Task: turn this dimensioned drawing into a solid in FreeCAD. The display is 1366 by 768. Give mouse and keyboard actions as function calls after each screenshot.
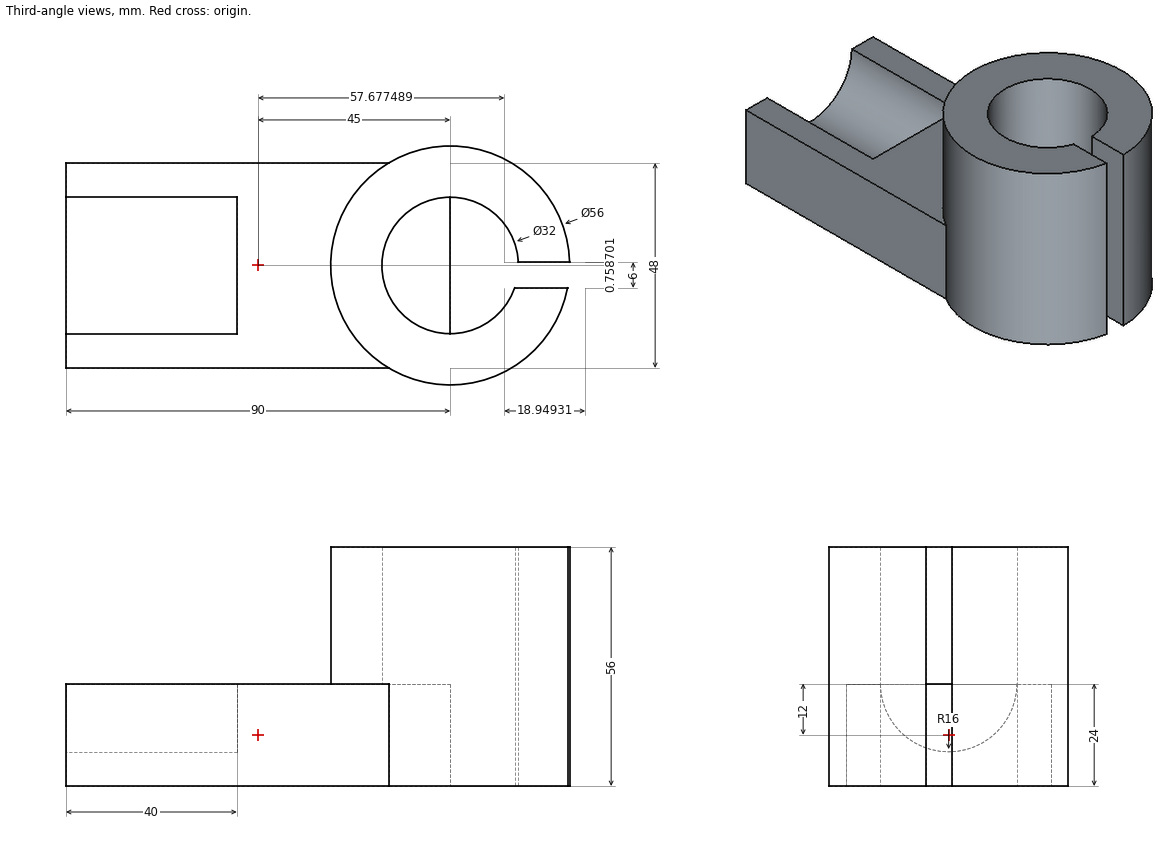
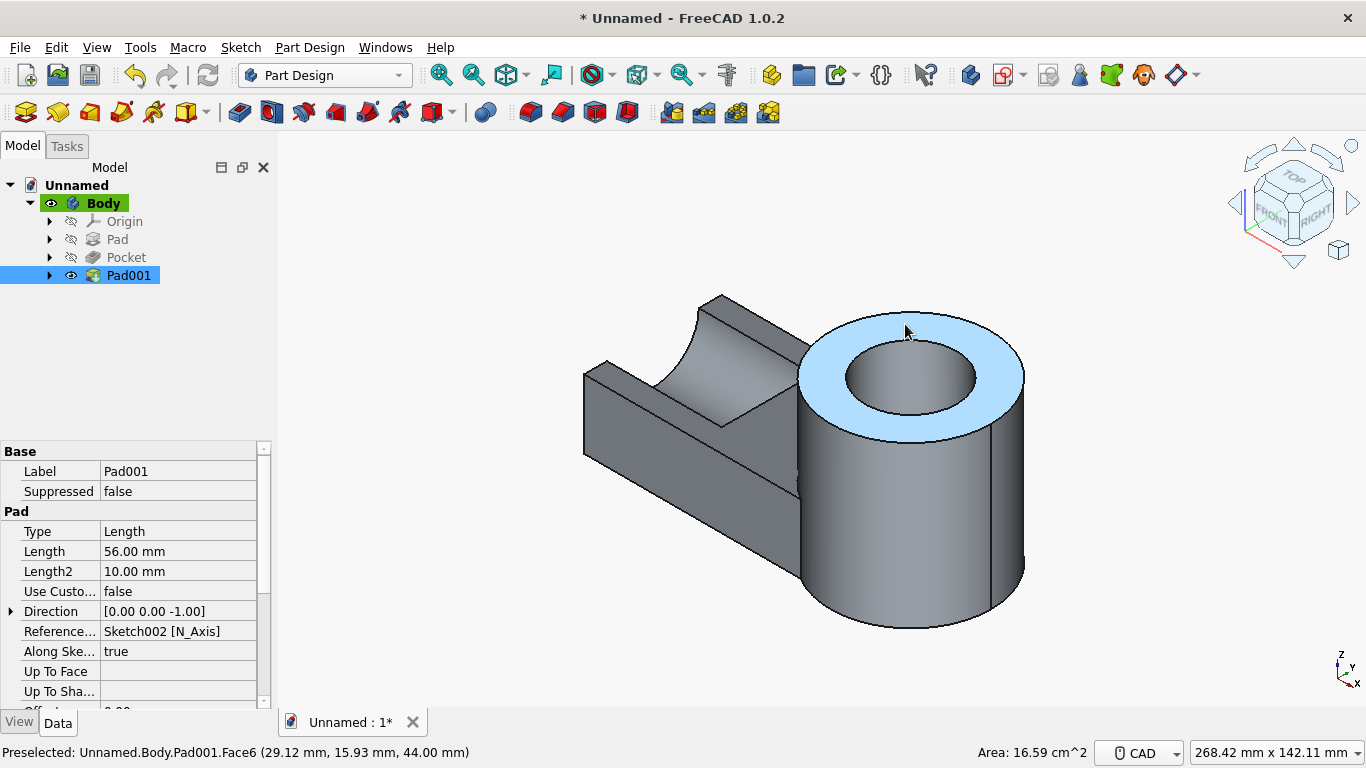
click(1004, 76)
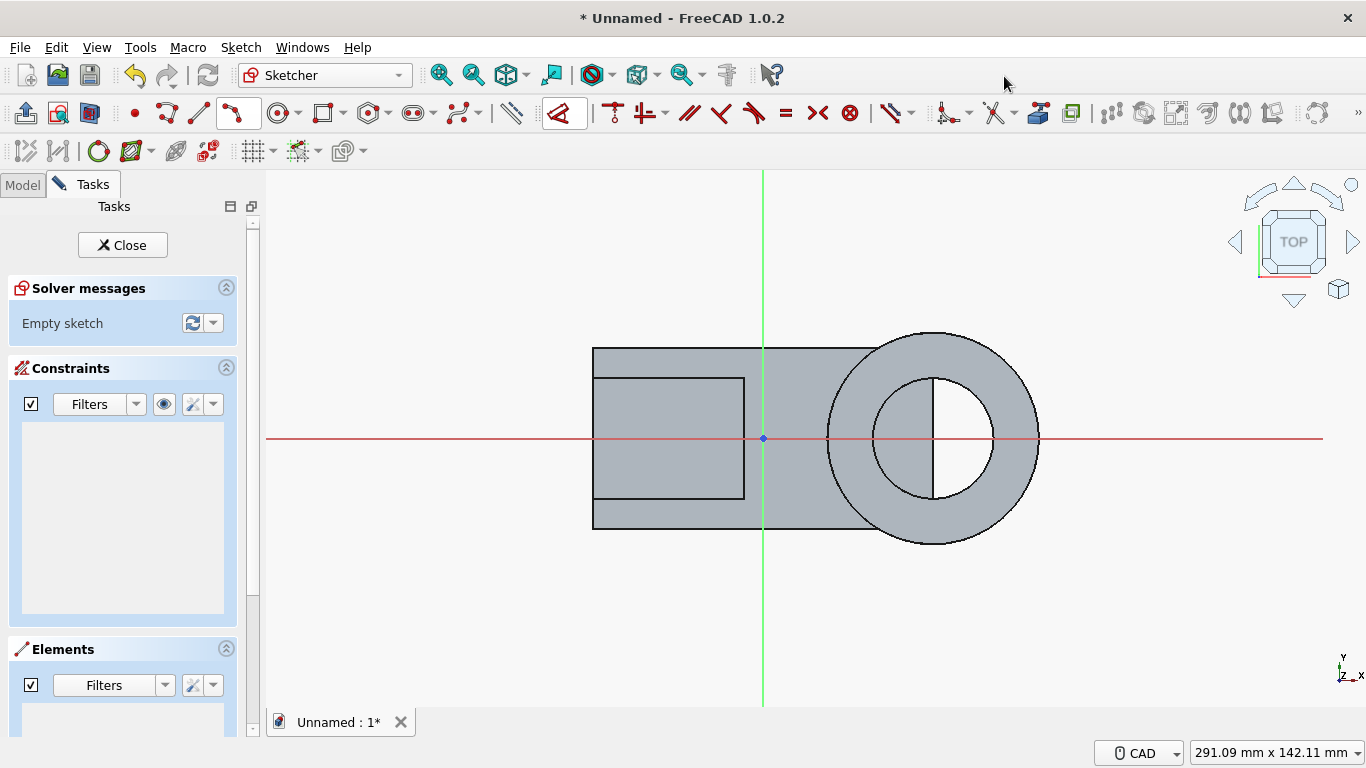
scroll(1050, 448, up, 11)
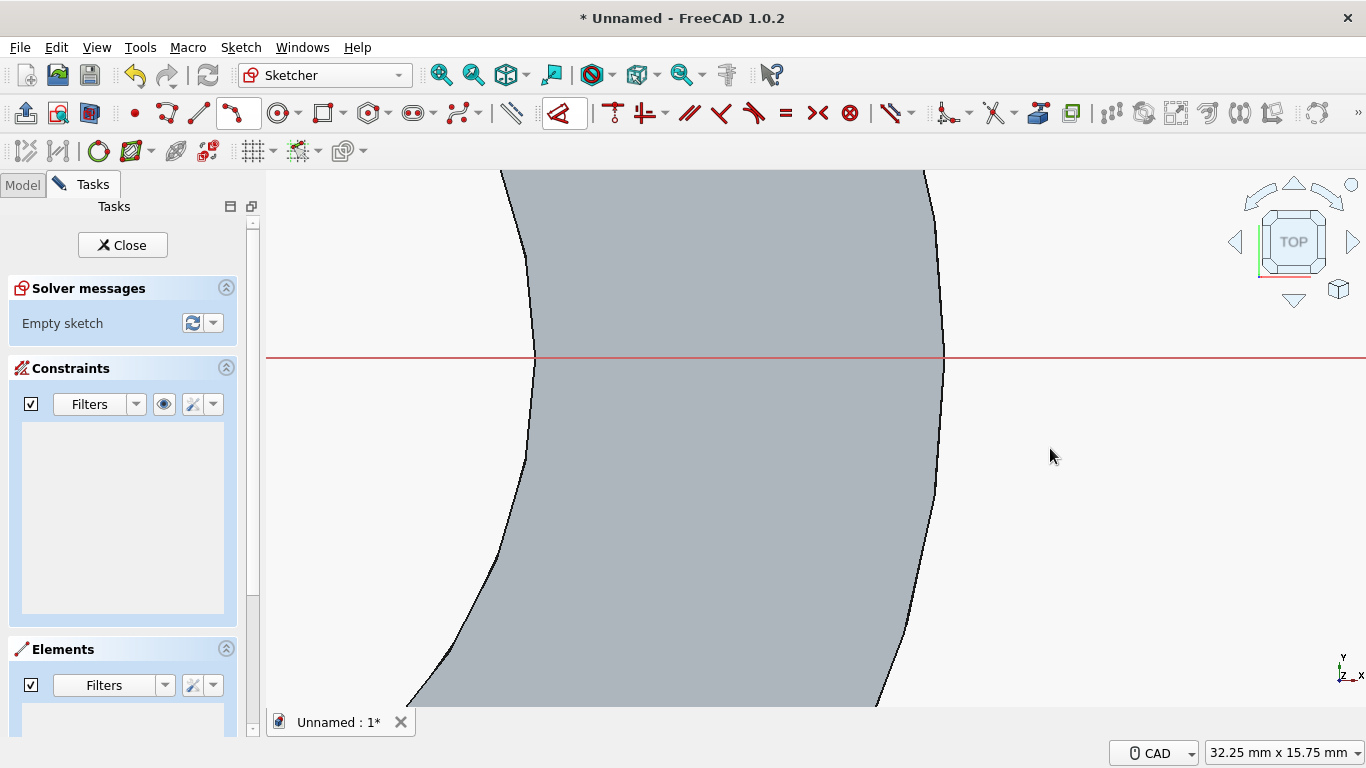
key(g)
key(r)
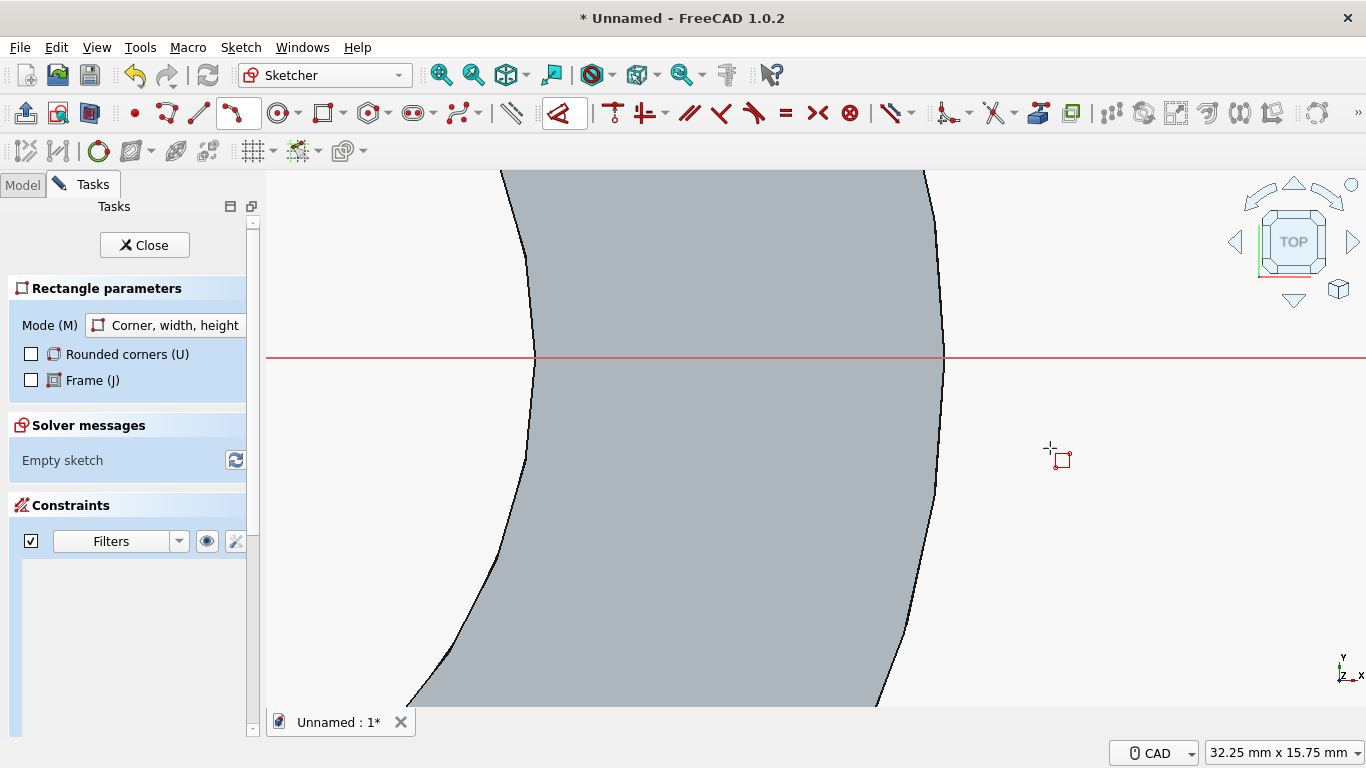
click(422, 332)
move(1068, 537)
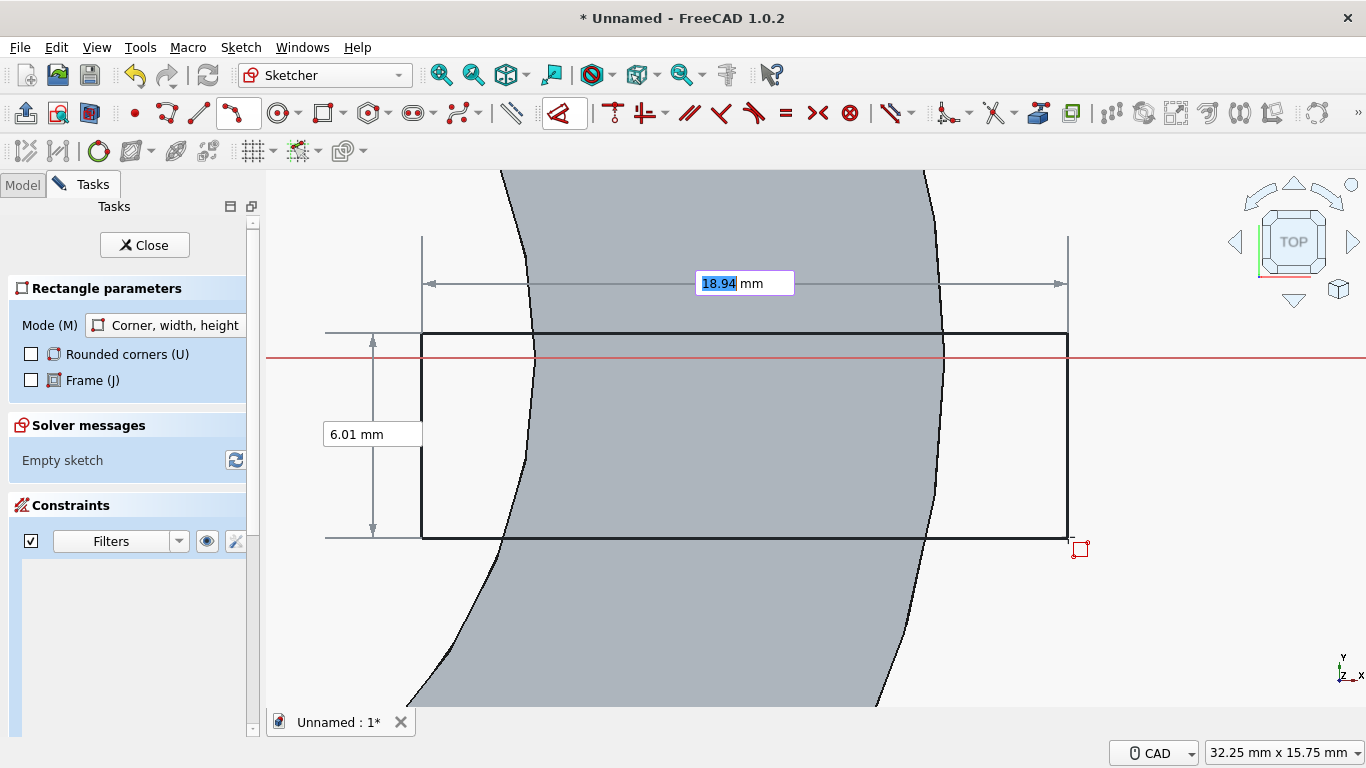
text(18.94931)
key(Tab)
text(6)
key(Return)
key(Escape)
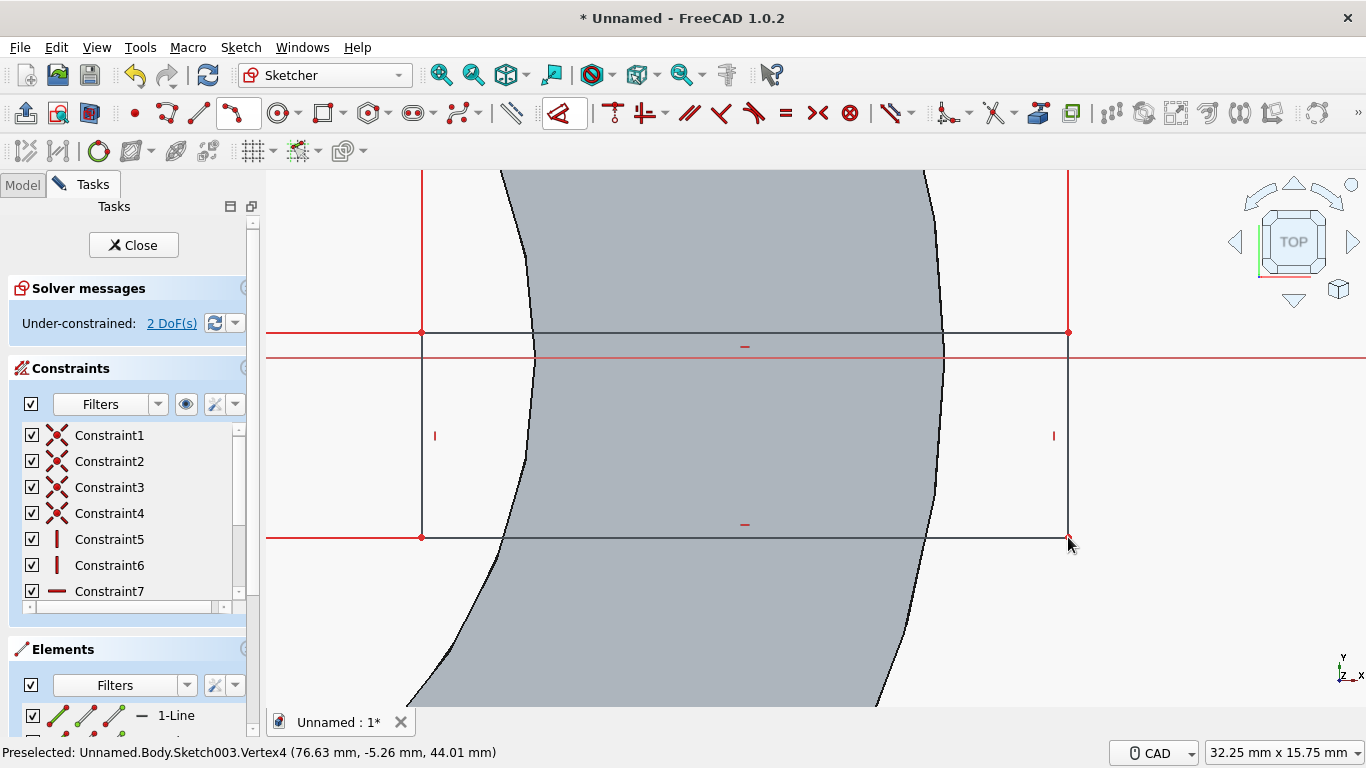
click(558, 114)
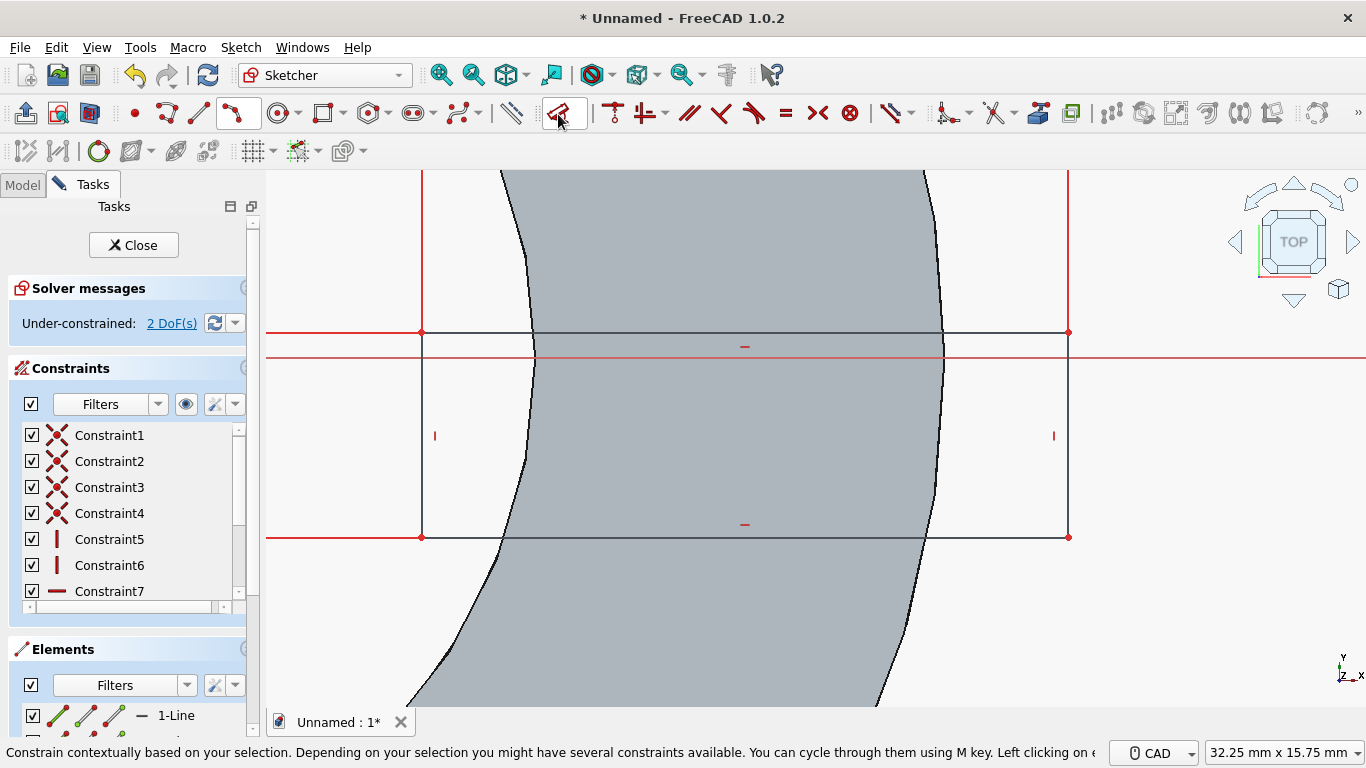
scroll(422, 333, up, 3)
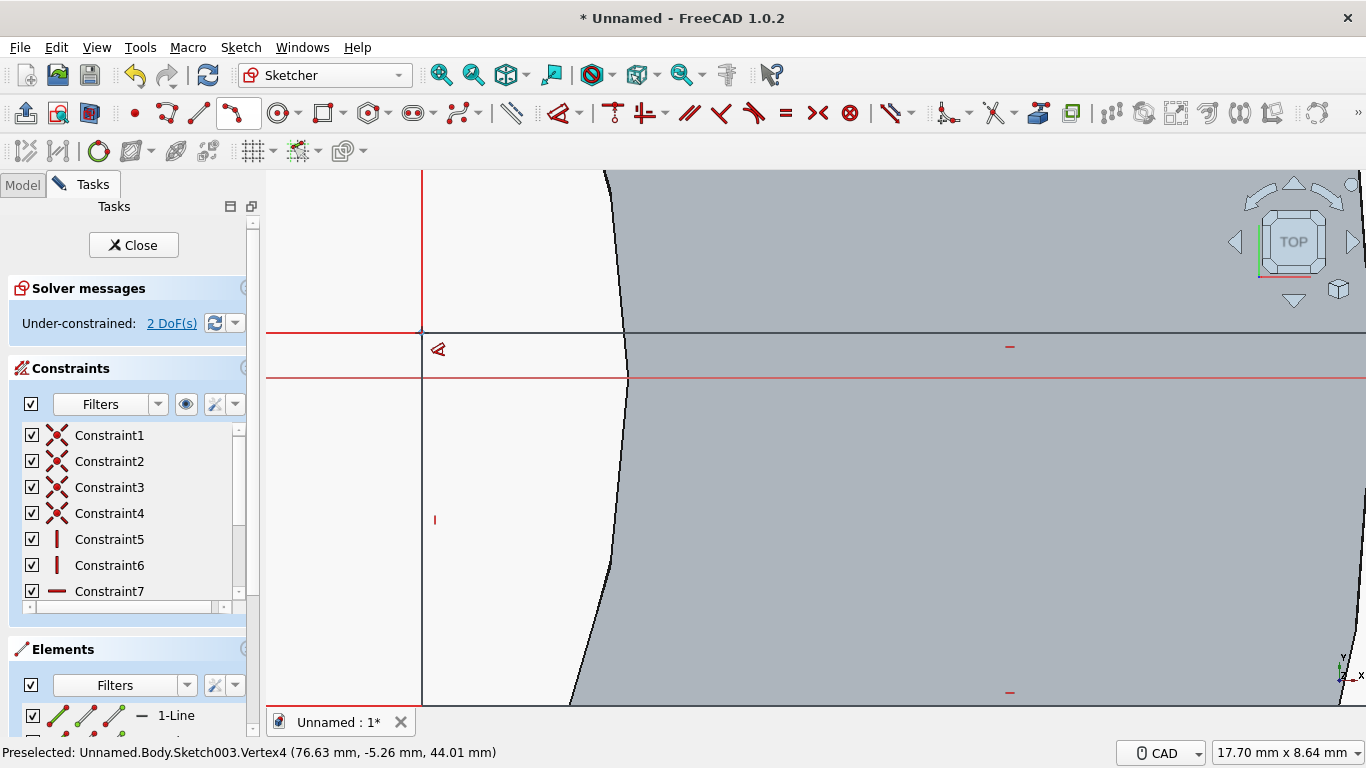
click(422, 333)
click(456, 356)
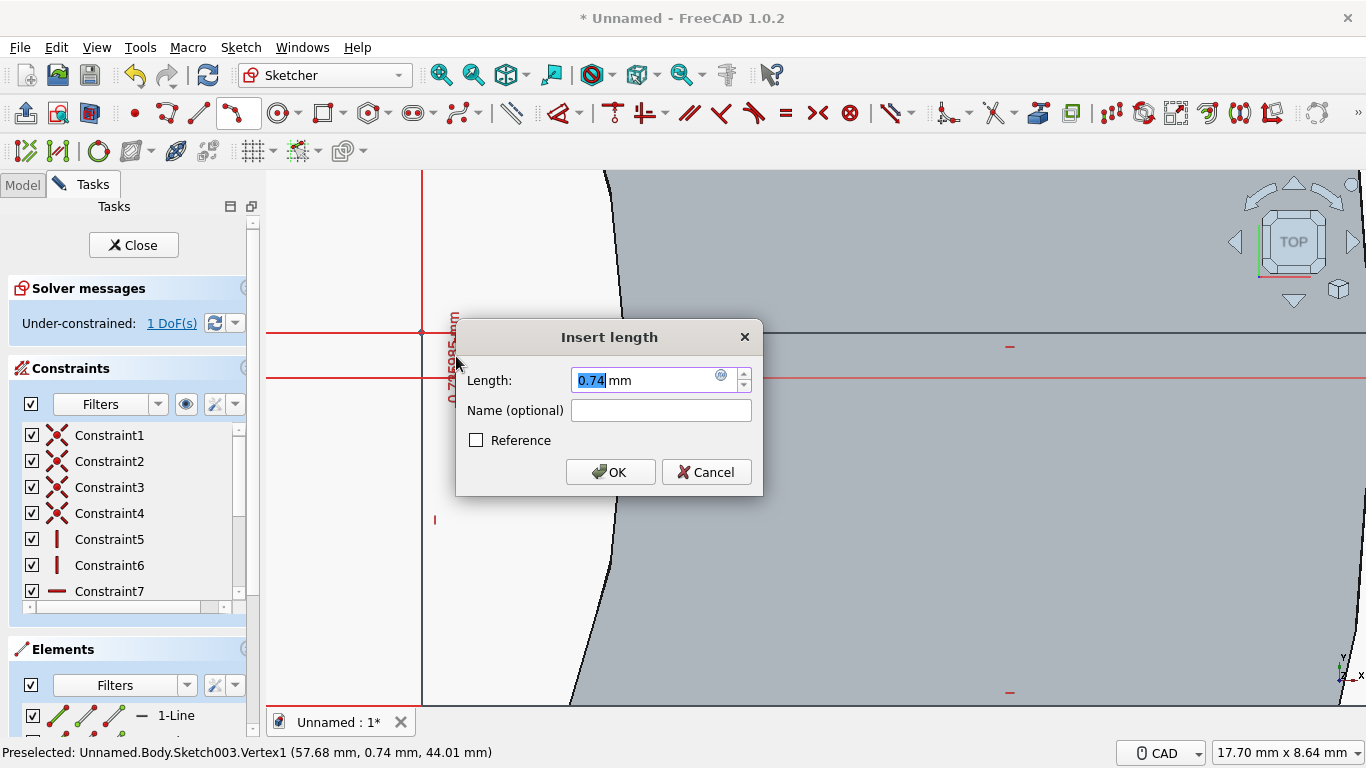
text(0.758701)
key(Return)